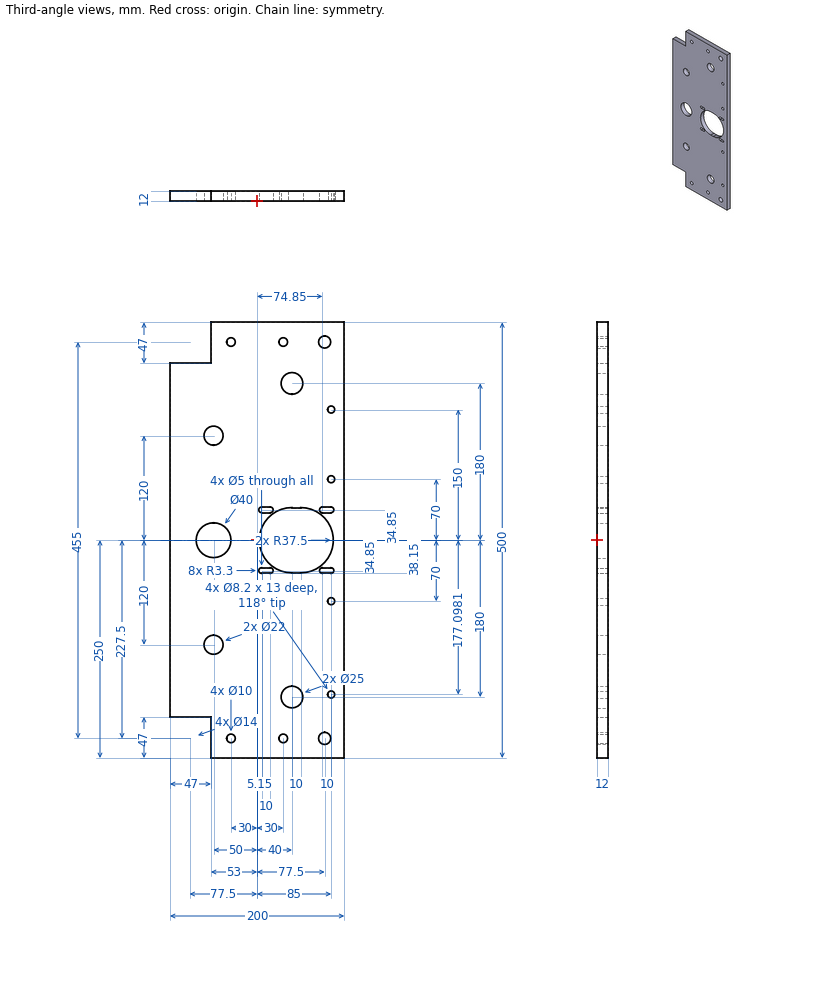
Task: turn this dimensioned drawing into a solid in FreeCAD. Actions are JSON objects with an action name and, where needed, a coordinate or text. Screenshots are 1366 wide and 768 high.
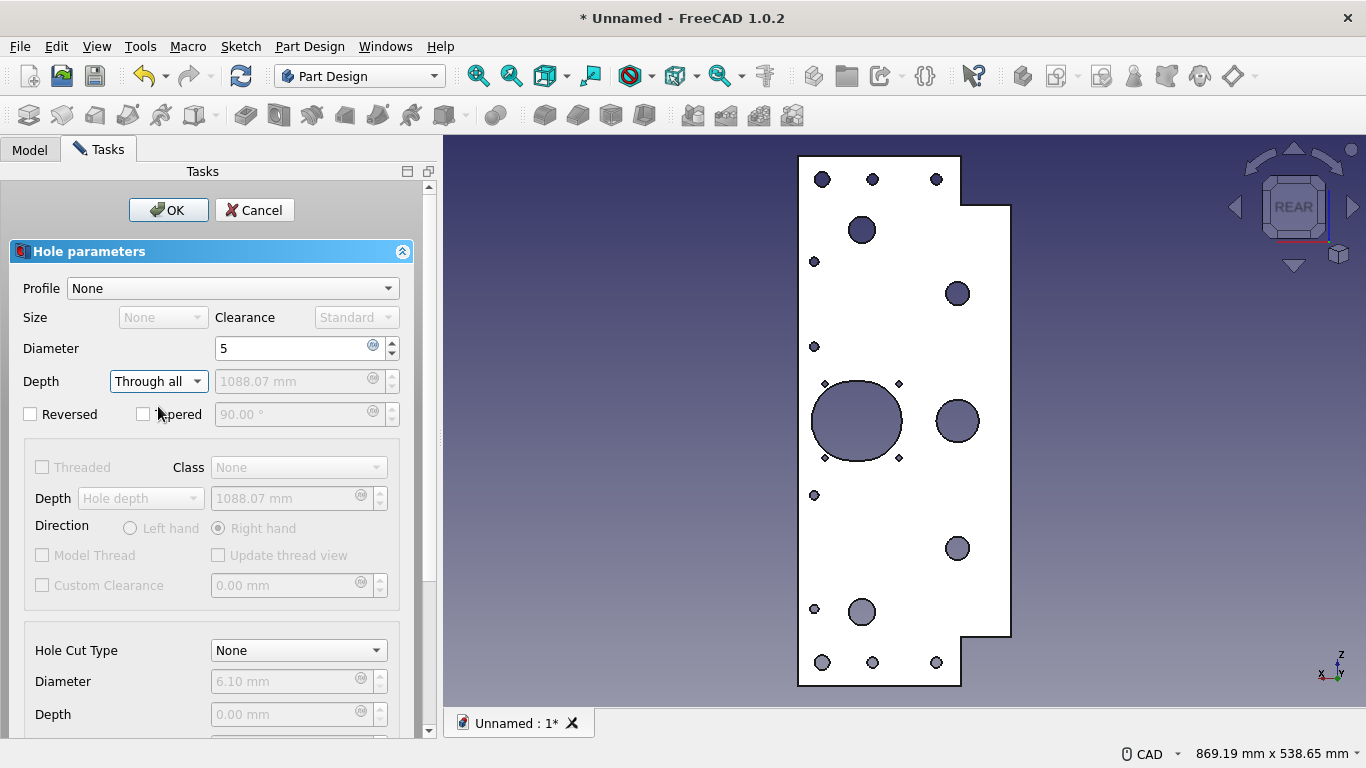
{"action": "left_click", "coordinate": [169, 210]}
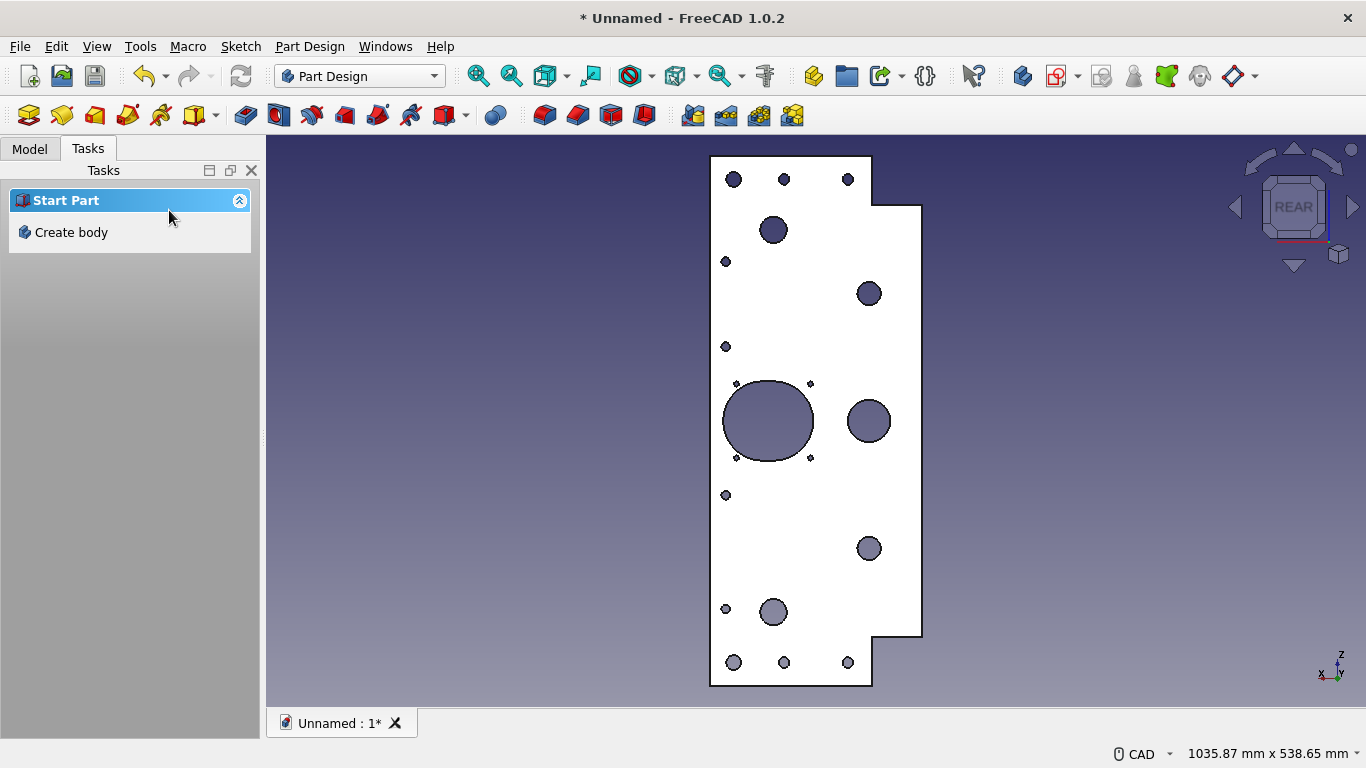
{"action": "left_click", "coordinate": [846, 496]}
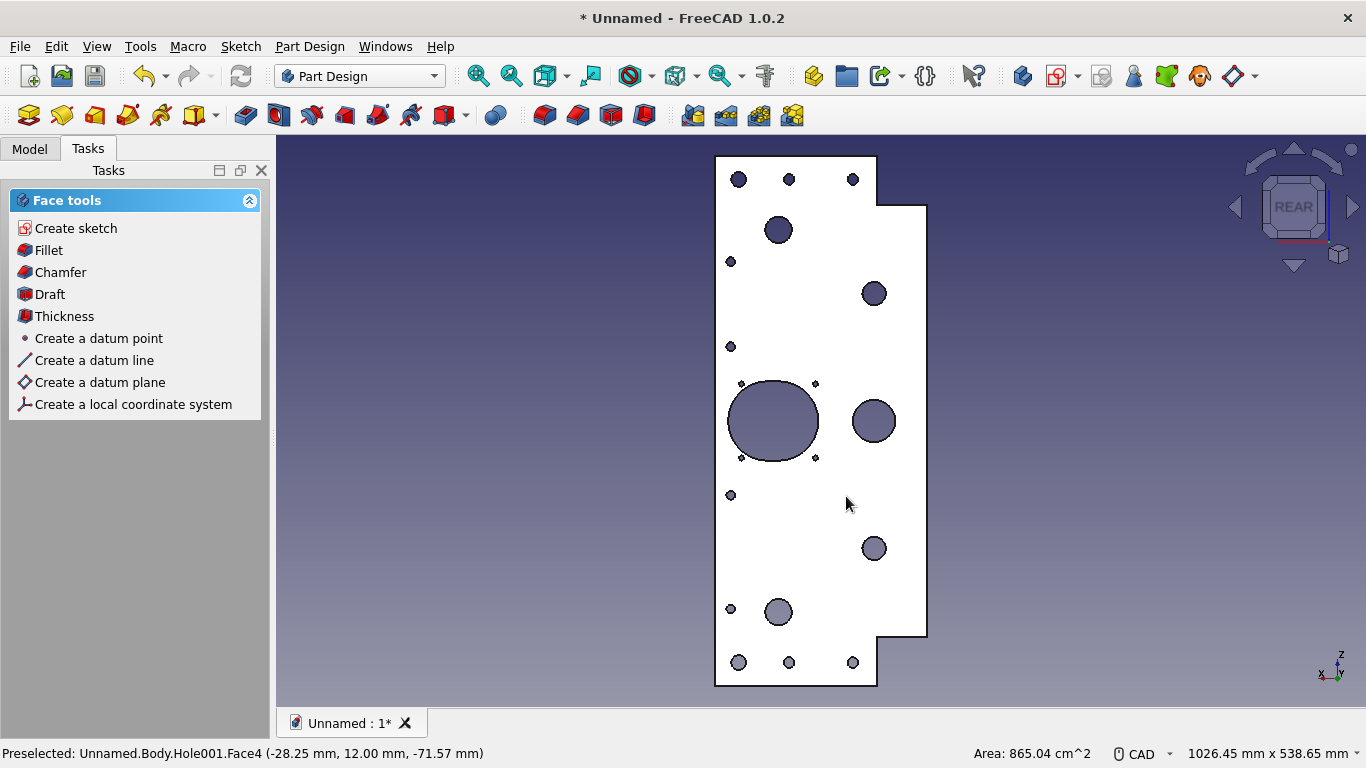
{"action": "left_click", "coordinate": [1056, 76]}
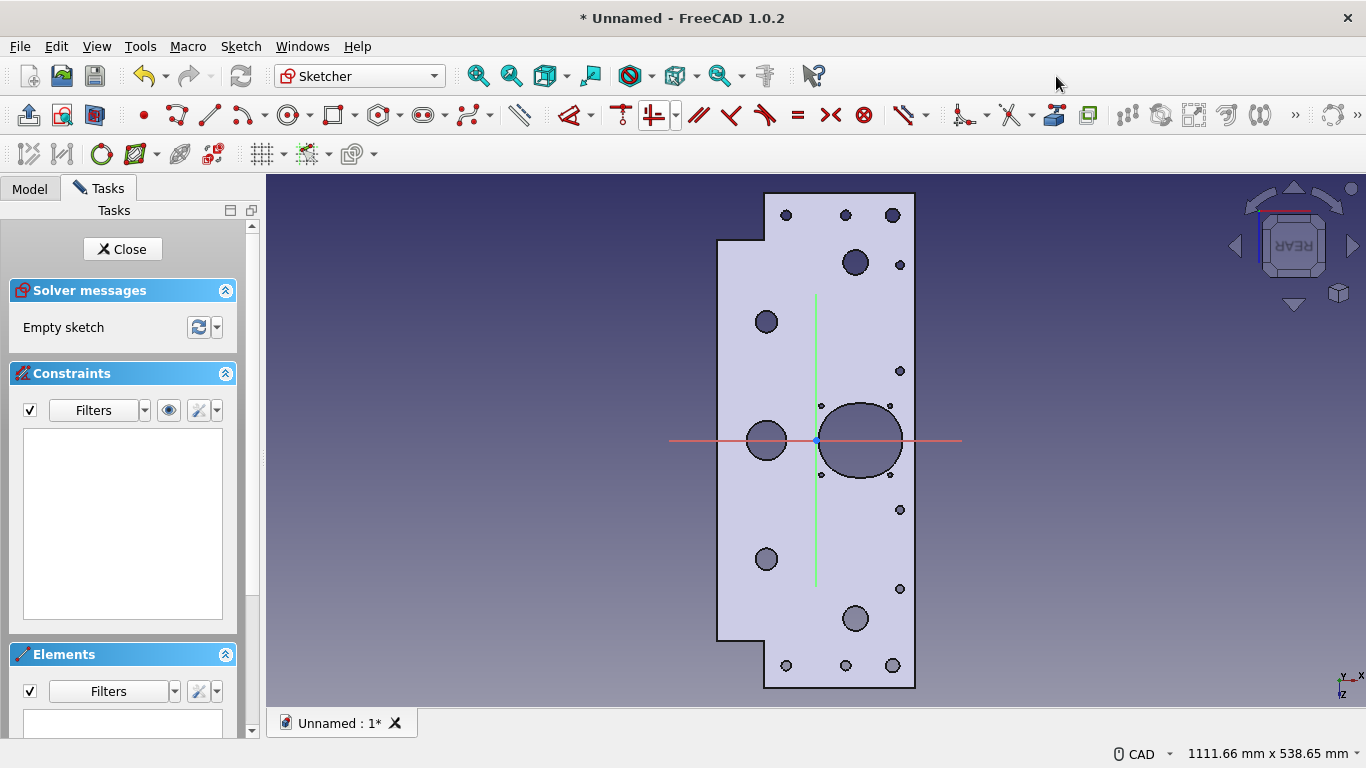
{"action": "scroll", "coordinate": [896, 440], "scroll_direction": "up", "scroll_amount": 7}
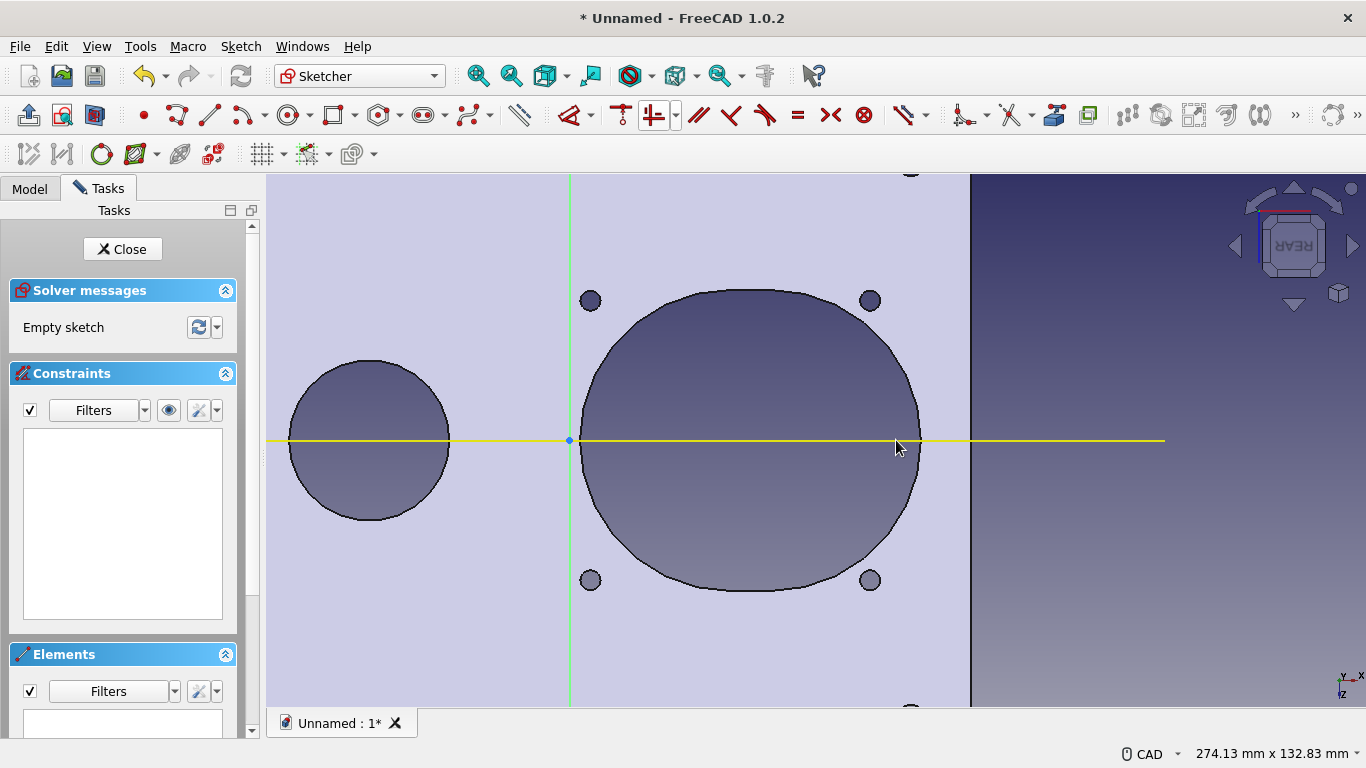
{"action": "left_click", "coordinate": [422, 116]}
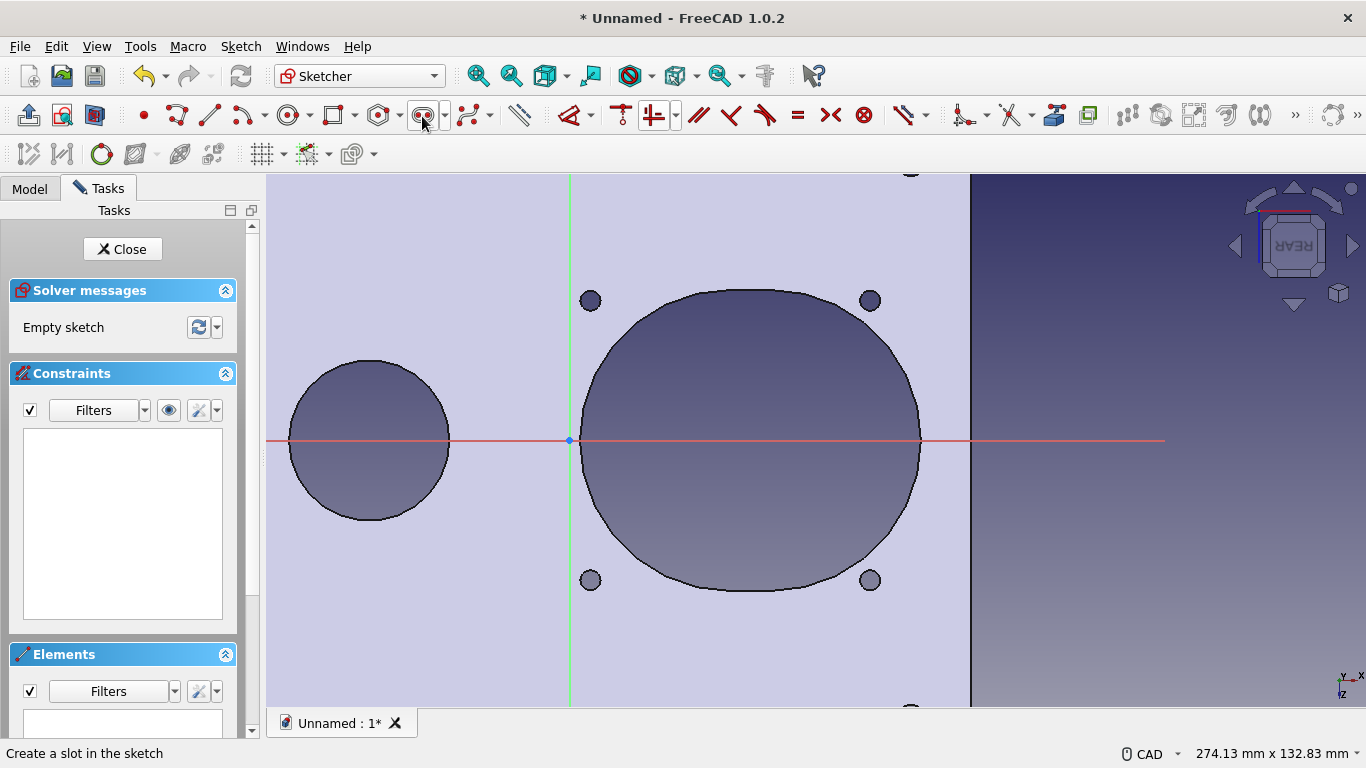
{"action": "scroll", "coordinate": [590, 301], "scroll_direction": "up", "scroll_amount": 3}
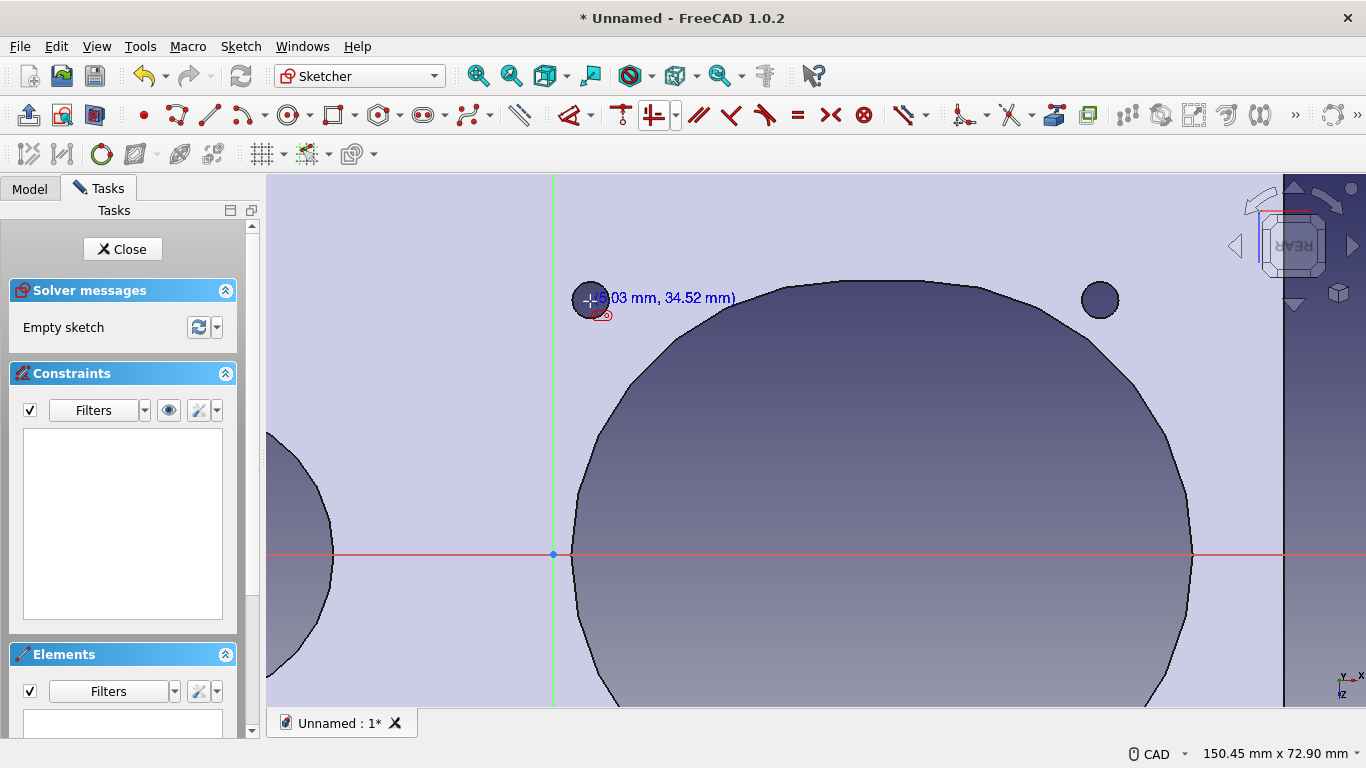
{"action": "left_click", "coordinate": [591, 300]}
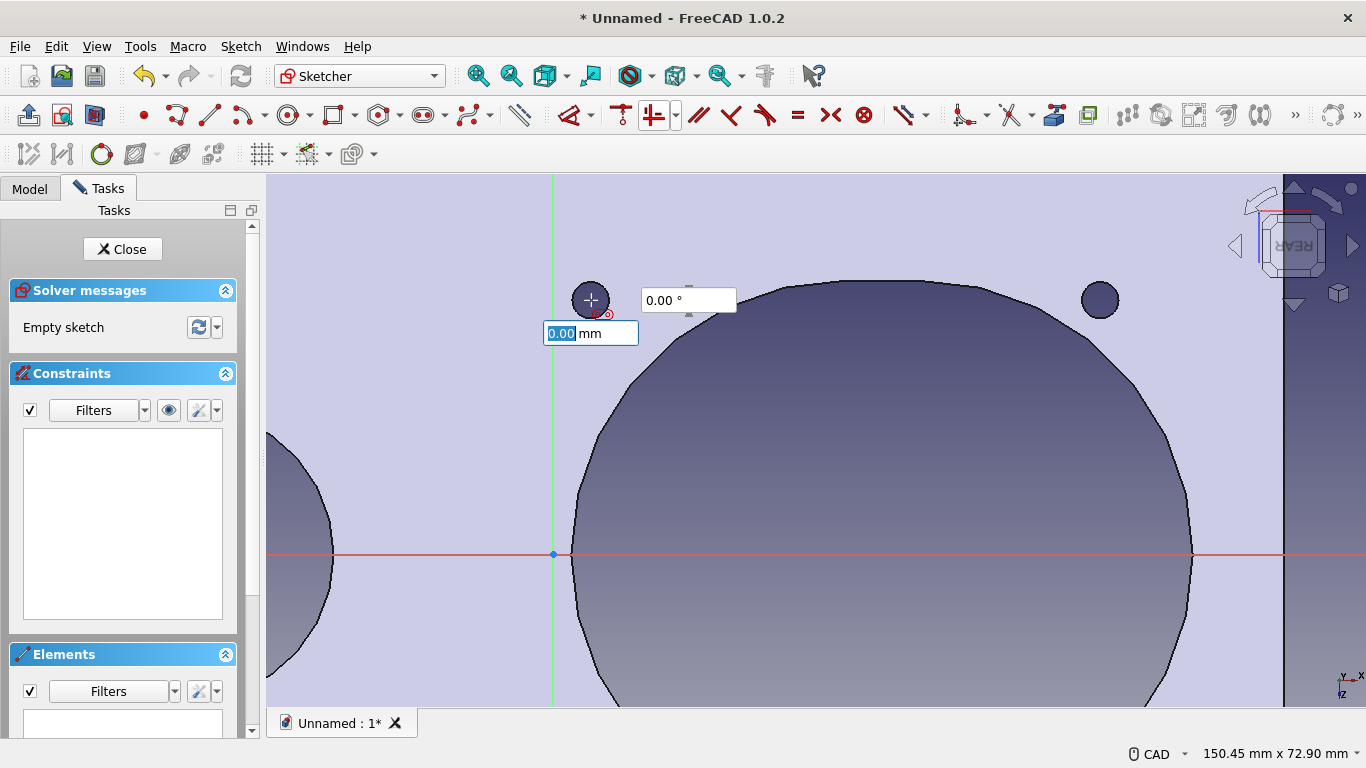
{"action": "left_click", "coordinate": [664, 300]}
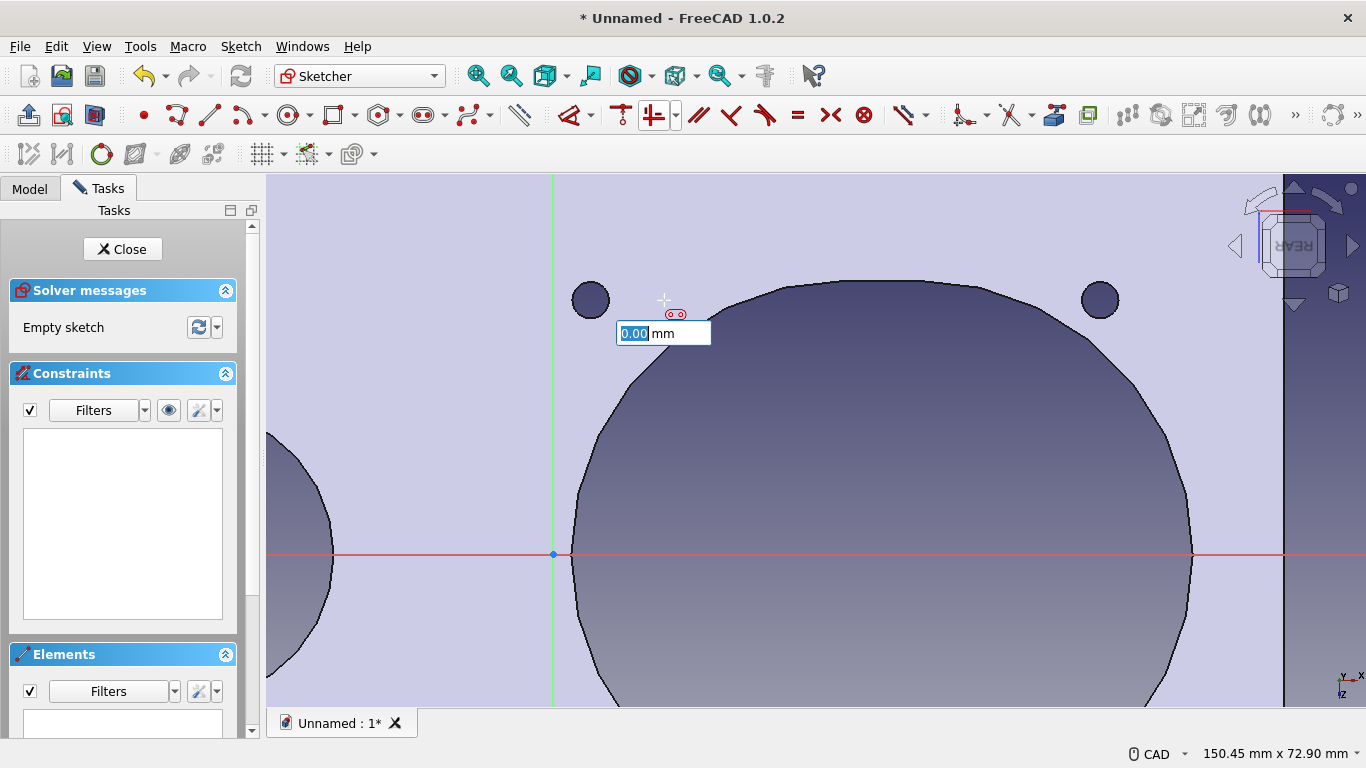
{"action": "left_click", "coordinate": [627, 276]}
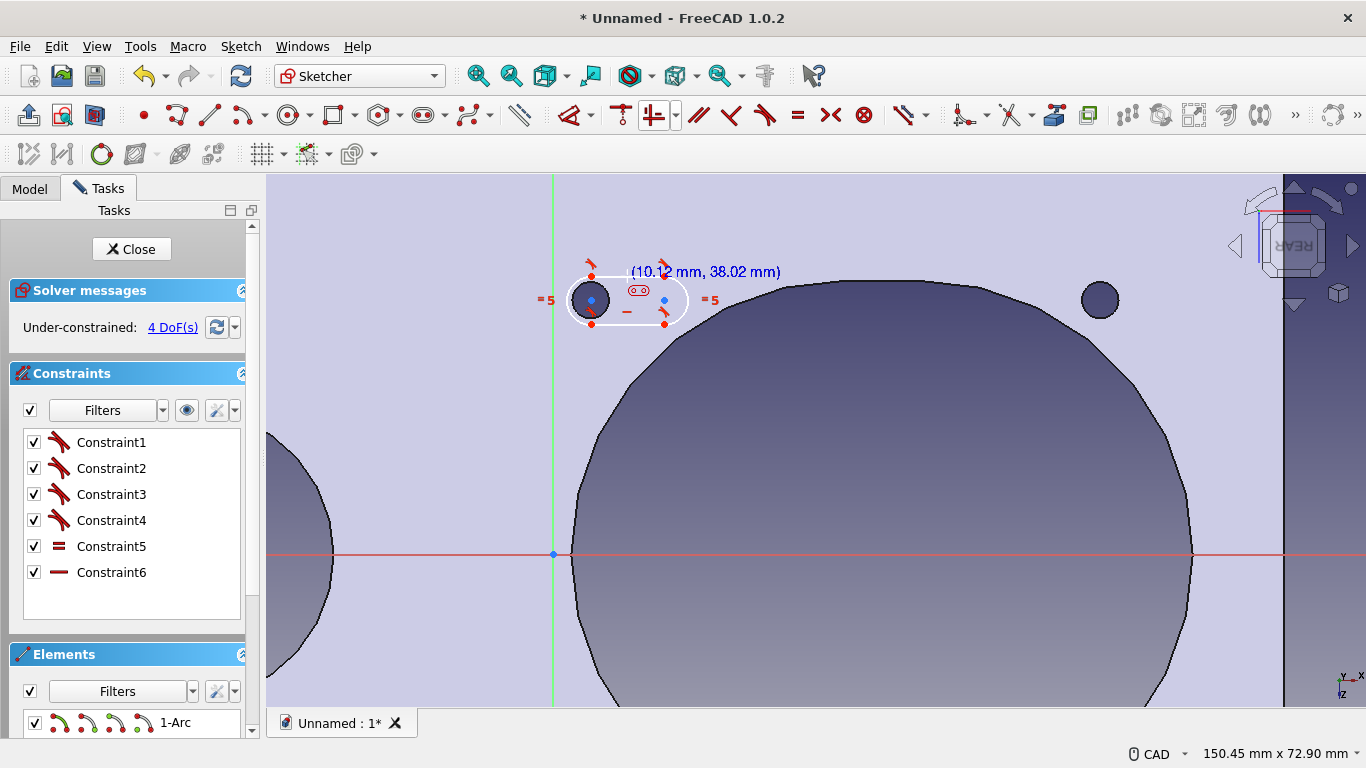
{"action": "left_click", "coordinate": [1100, 300]}